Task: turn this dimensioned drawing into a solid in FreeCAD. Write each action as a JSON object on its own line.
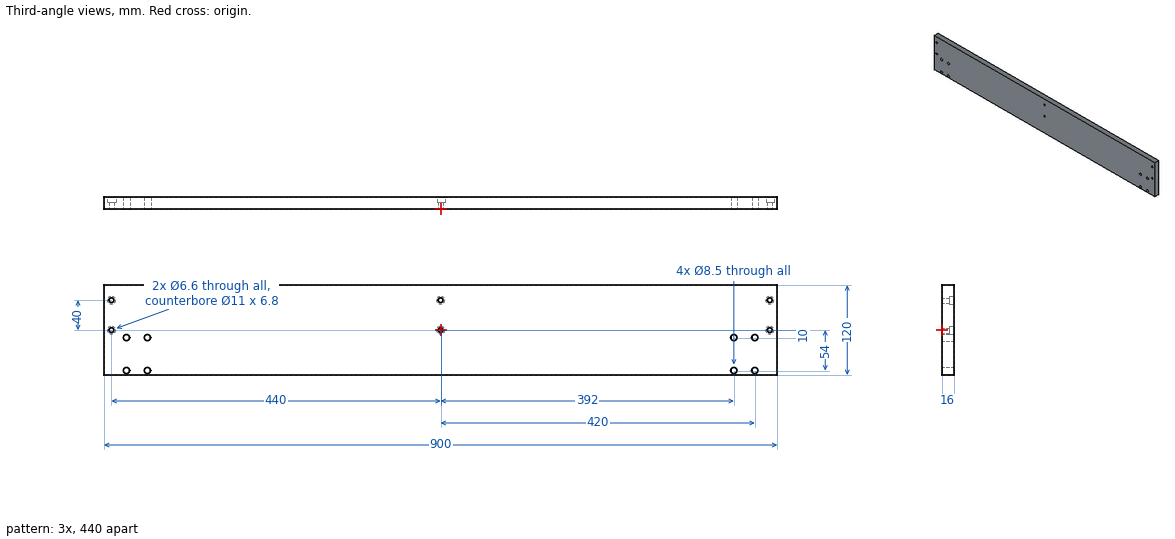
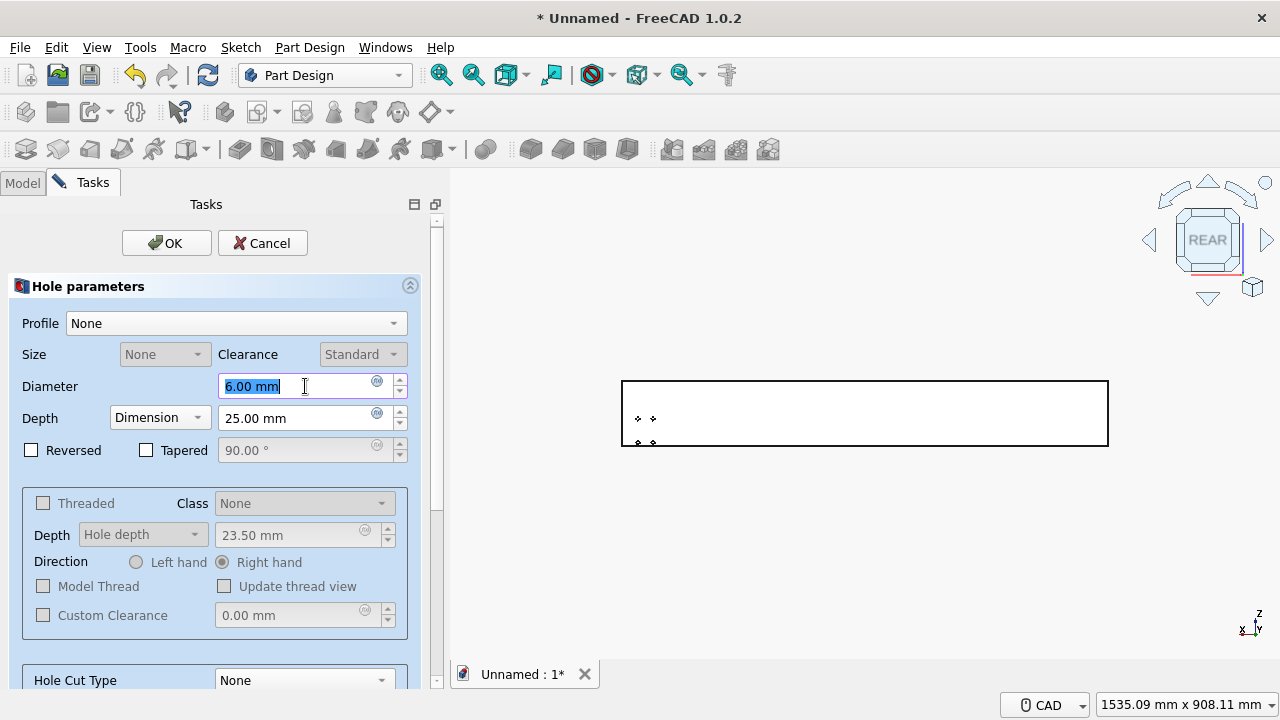
{"action": "type", "text": "8.5"}
{"action": "key", "text": "Tab"}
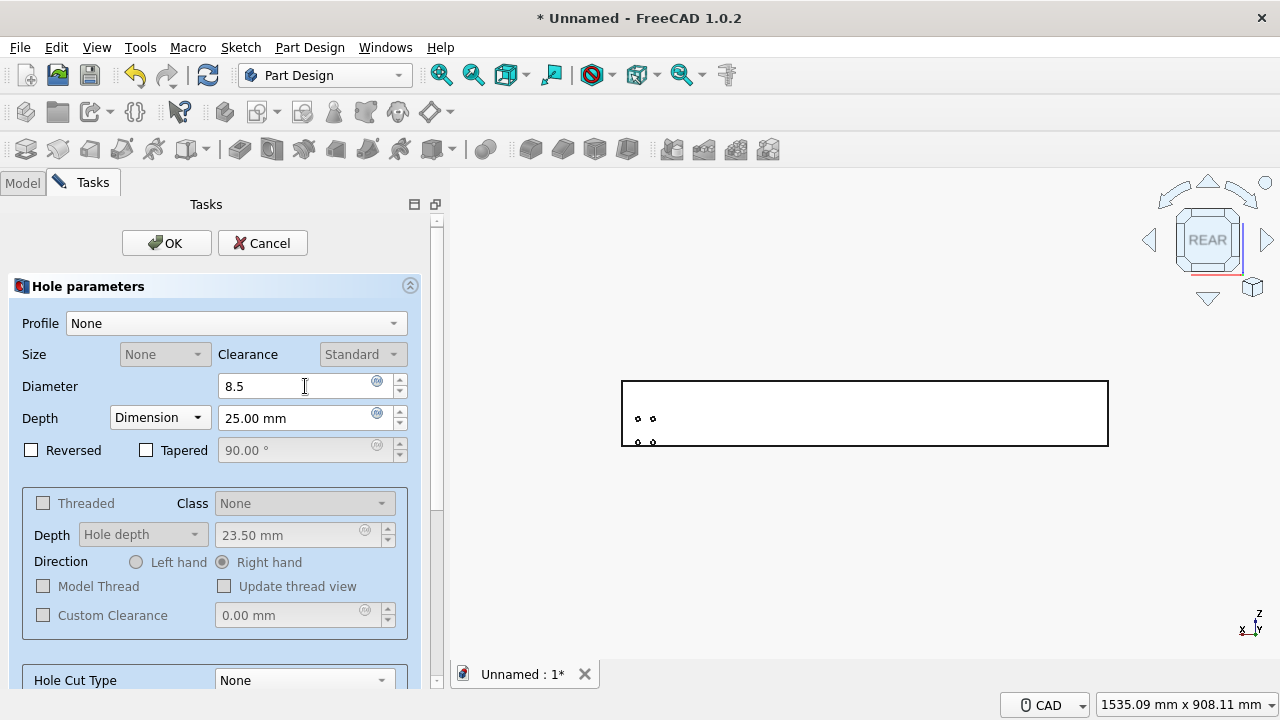
{"action": "left_click", "coordinate": [161, 418]}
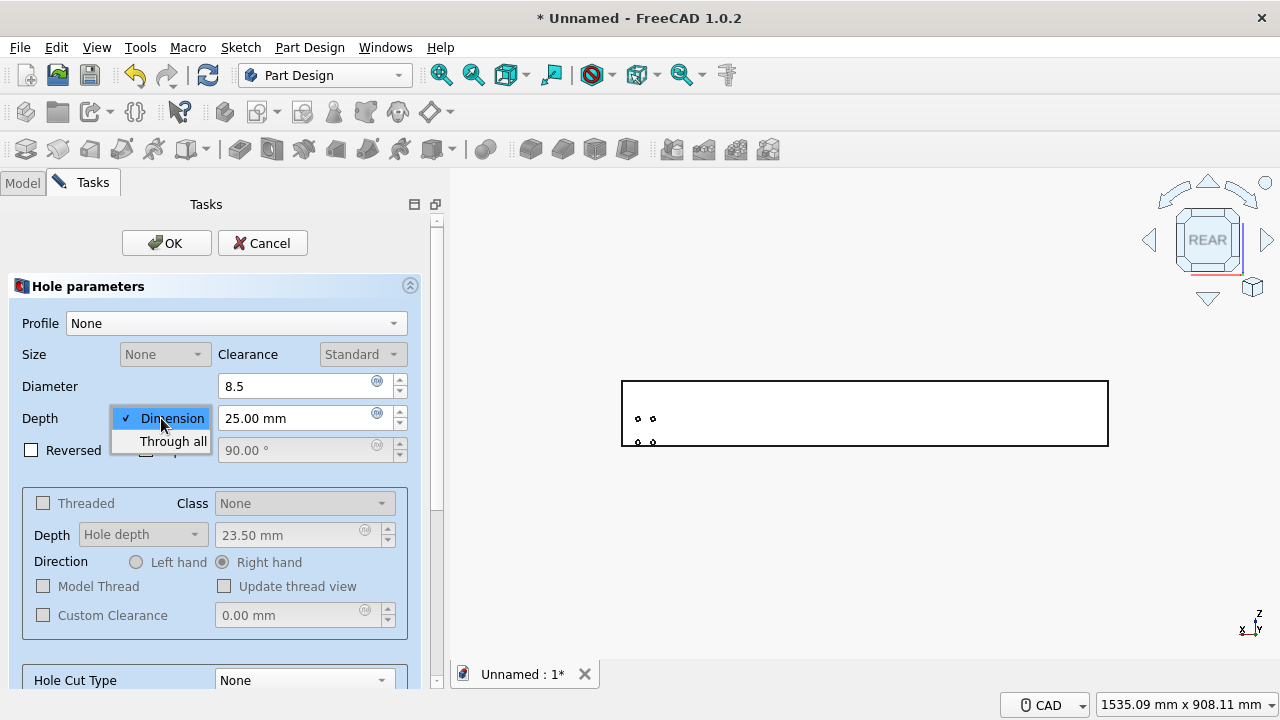
{"action": "left_click", "coordinate": [160, 442]}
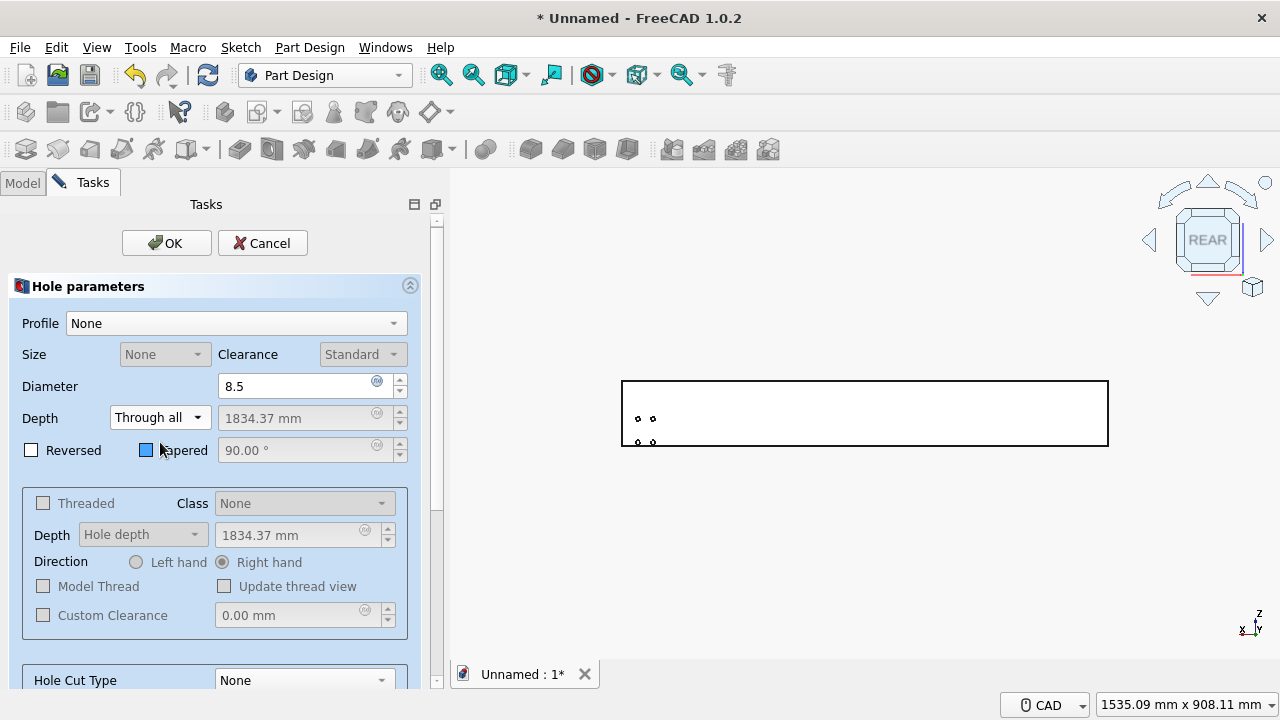
{"action": "left_click", "coordinate": [167, 243]}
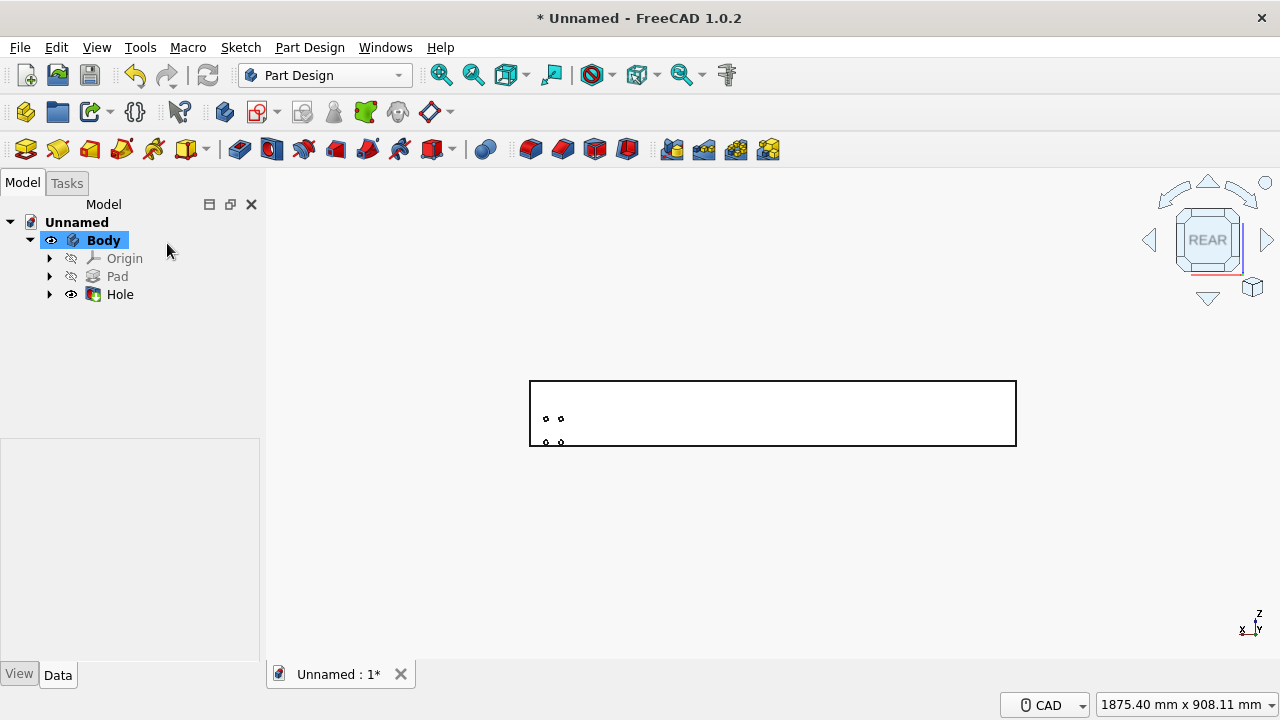
{"action": "left_click", "coordinate": [634, 413]}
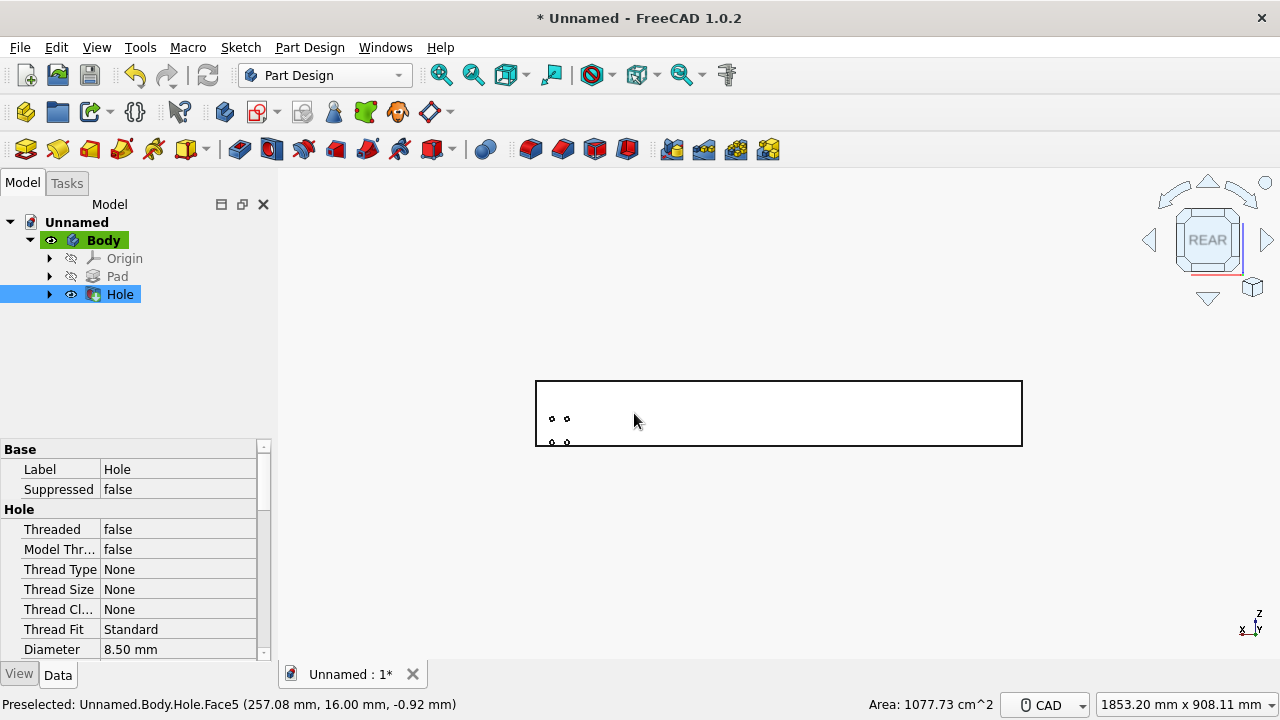
{"action": "left_click", "coordinate": [258, 112]}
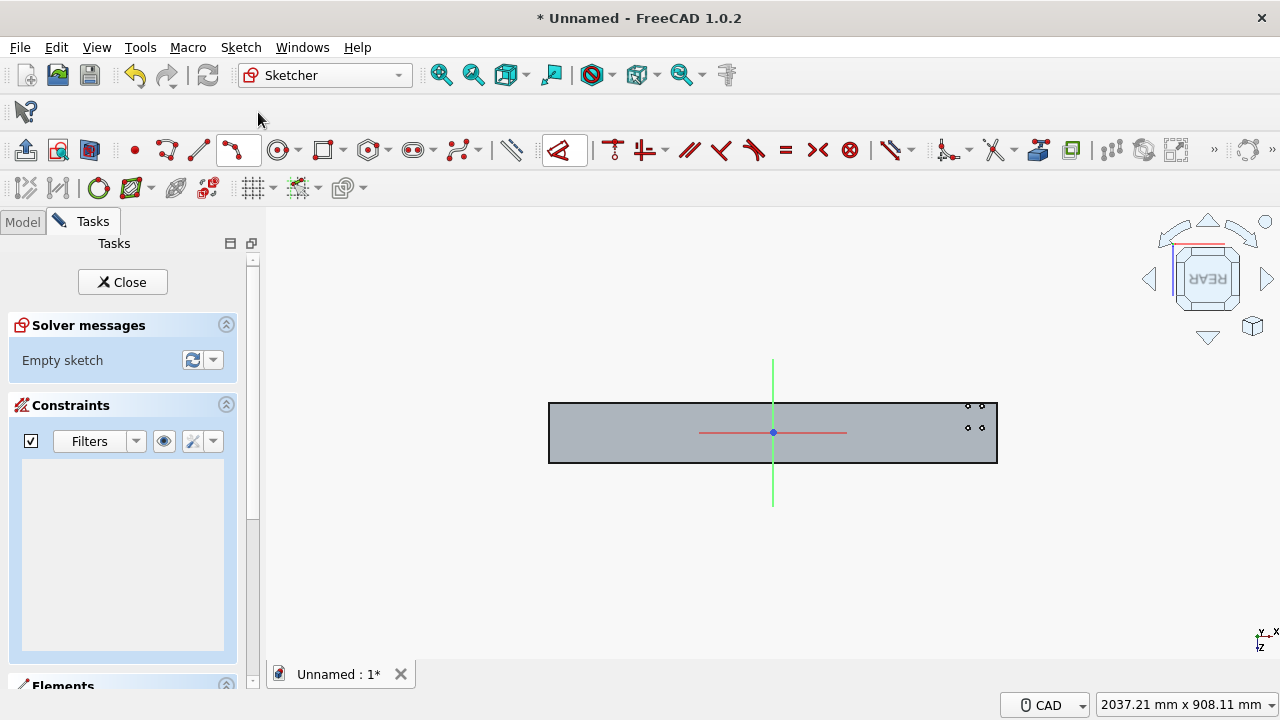
{"action": "scroll", "coordinate": [539, 444], "scroll_direction": "up", "scroll_amount": 12}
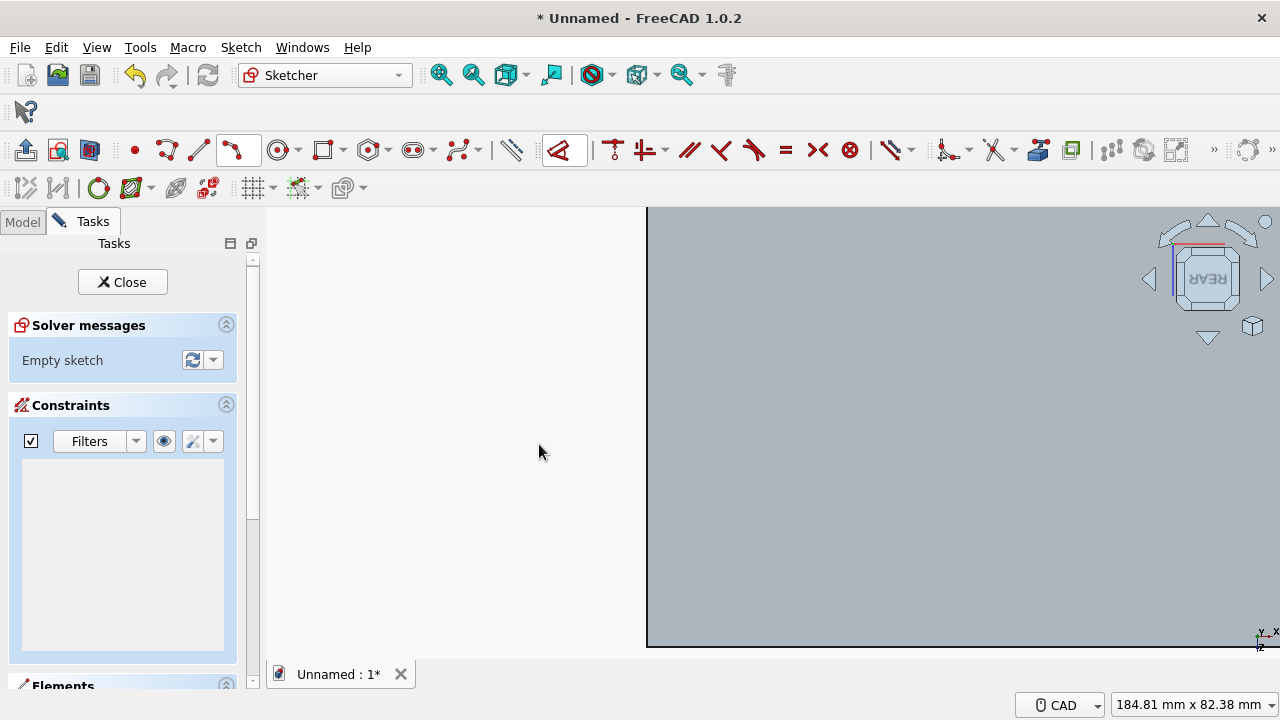
{"action": "key", "text": "g c"}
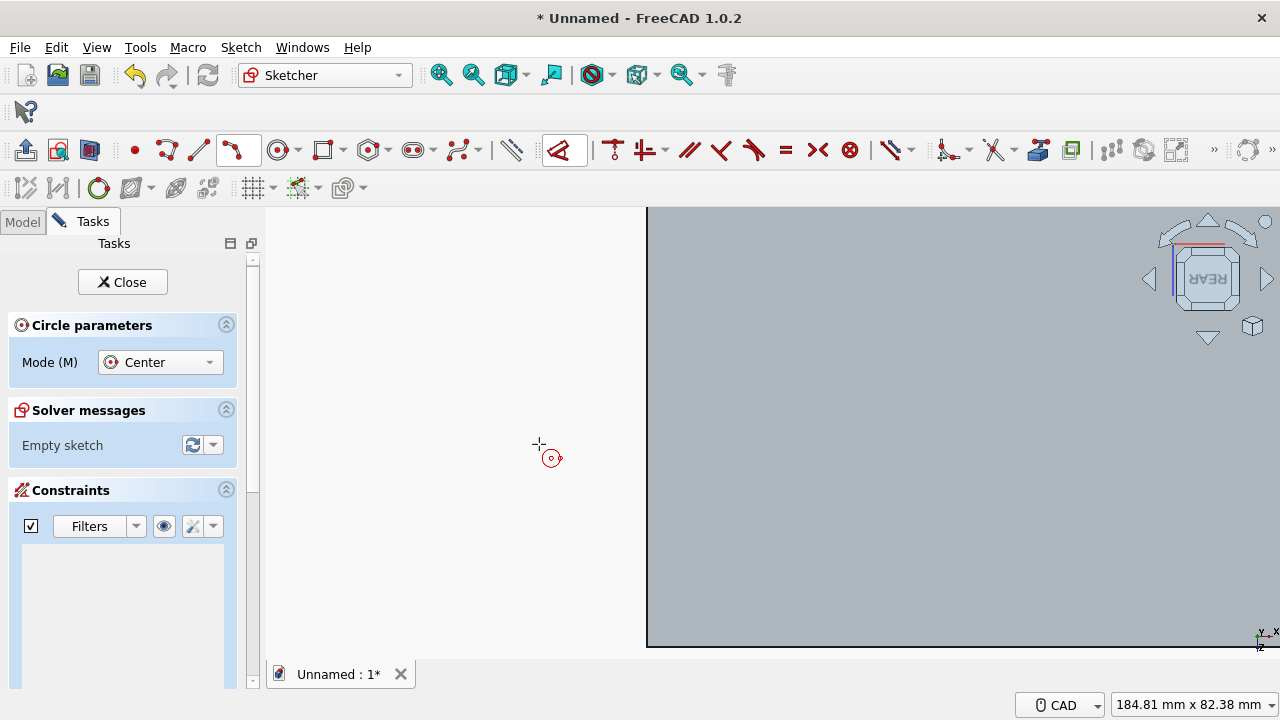
{"action": "scroll", "coordinate": [702, 317], "scroll_direction": "up", "scroll_amount": 2}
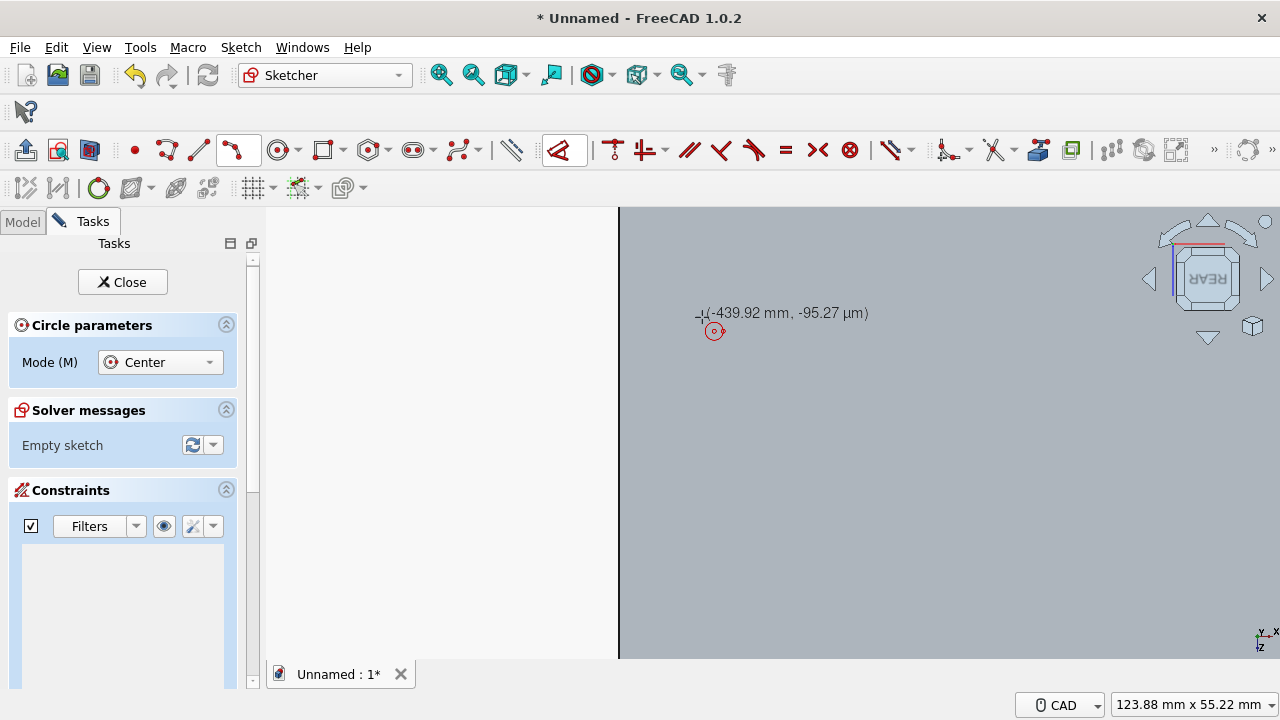
{"action": "left_click", "coordinate": [701, 318]}
{"action": "mouse_move", "coordinate": [720, 298]}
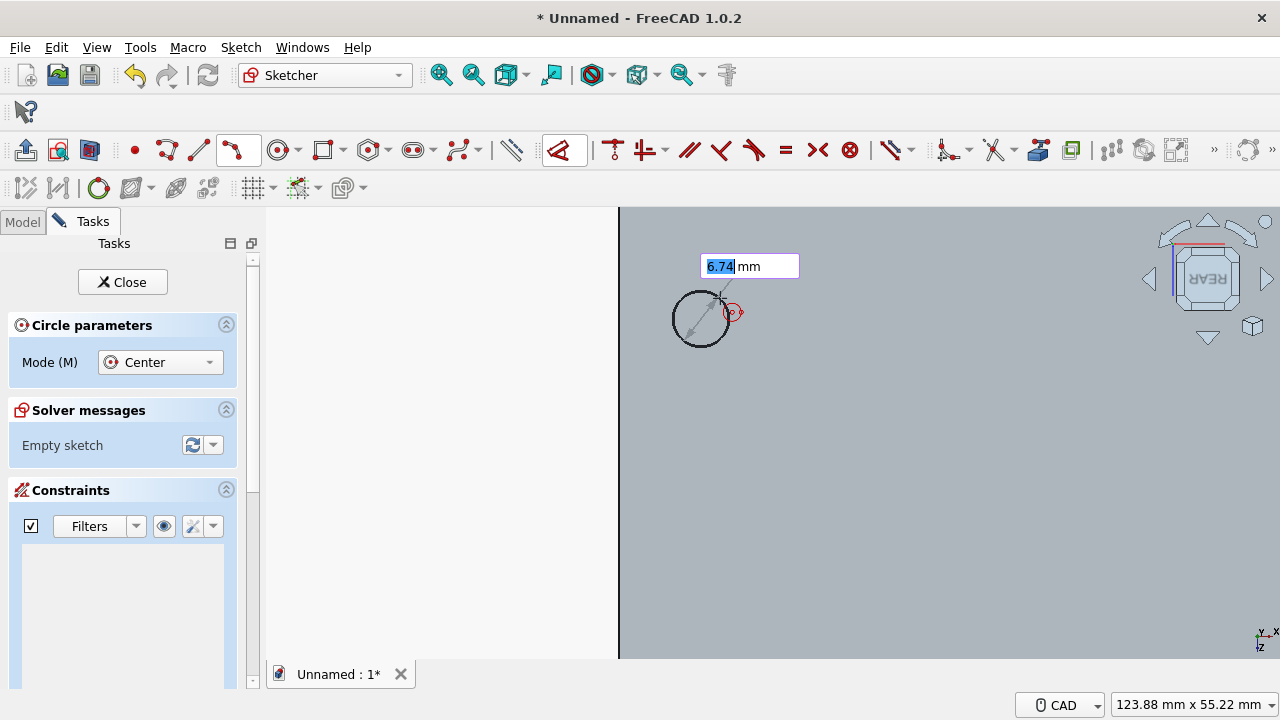
{"action": "type", "text": "6.6"}
{"action": "key", "text": "Return"}